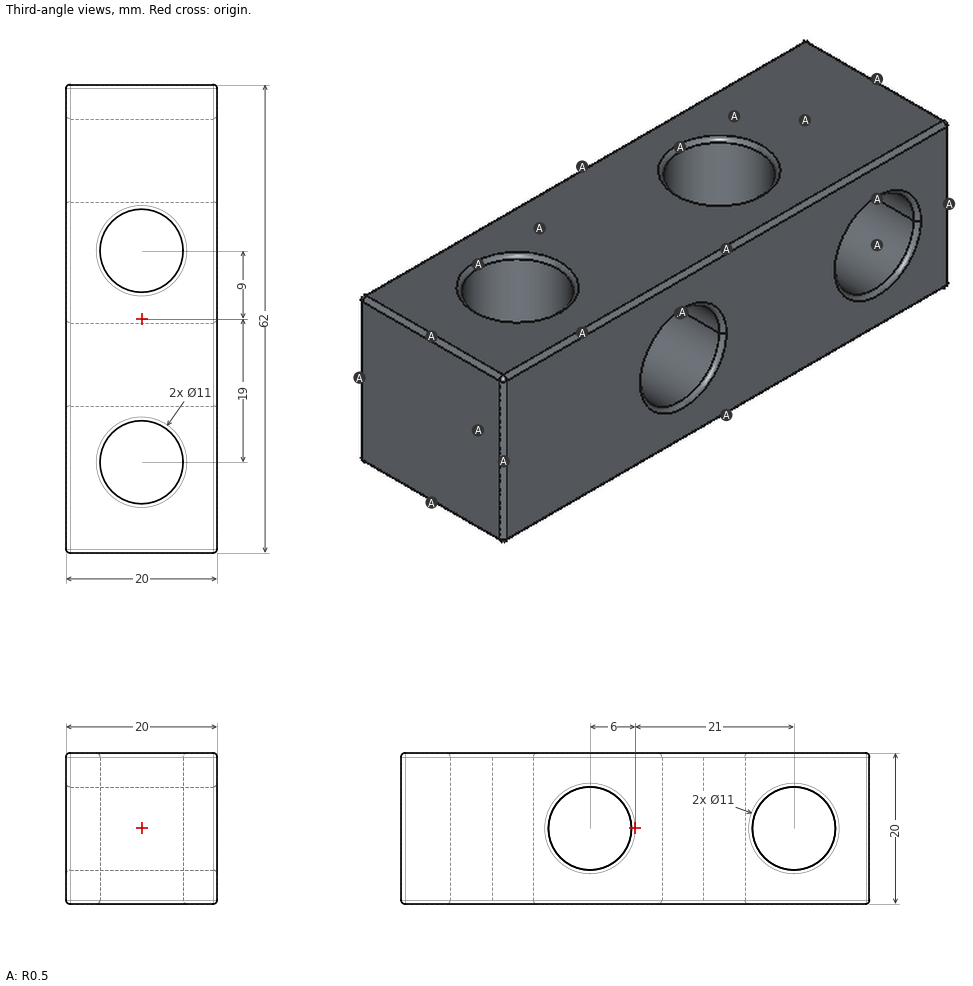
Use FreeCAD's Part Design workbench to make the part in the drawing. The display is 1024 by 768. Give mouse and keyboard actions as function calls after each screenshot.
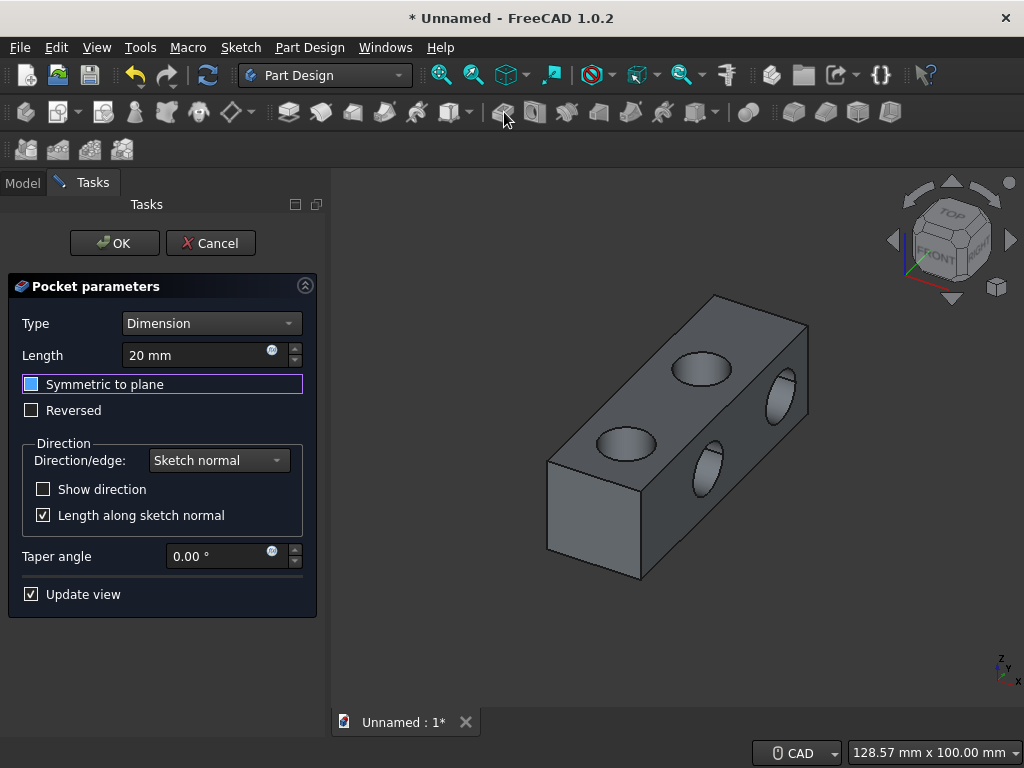
click(115, 243)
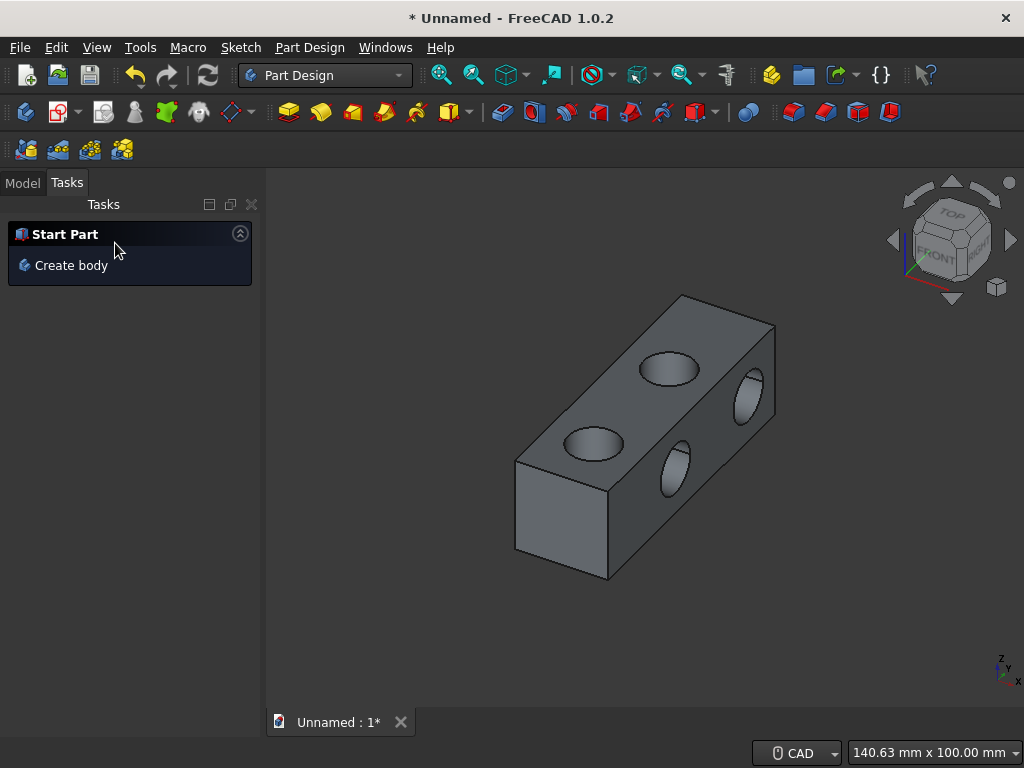
click(716, 416)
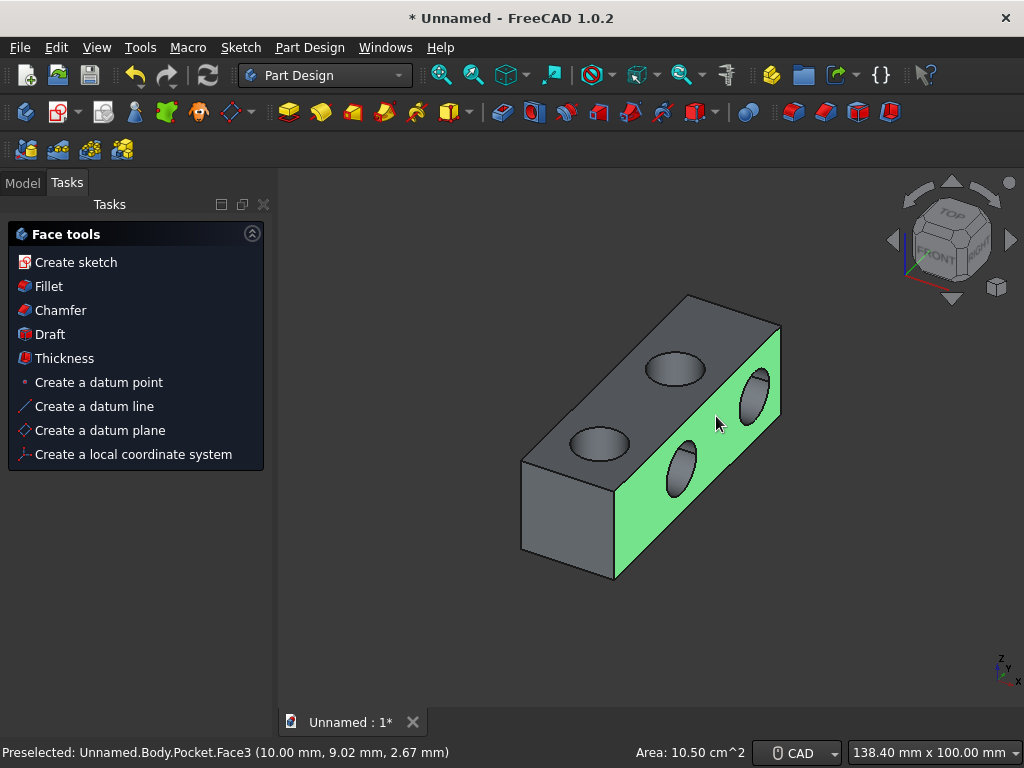
click(640, 420, ctrl)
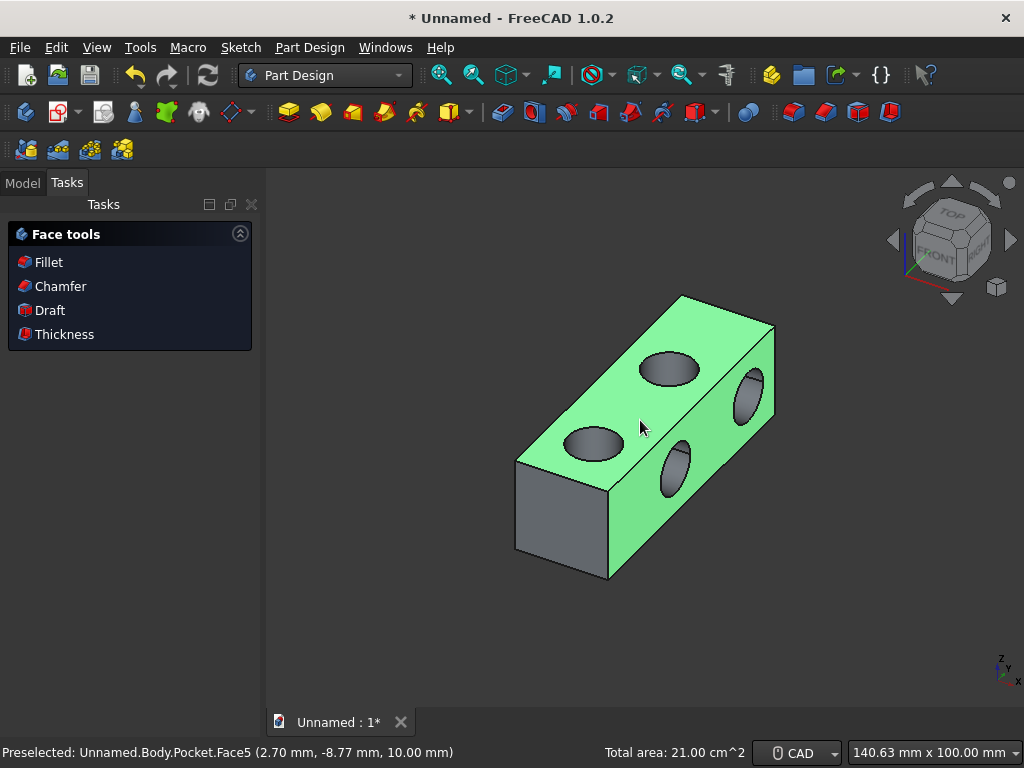
key(0)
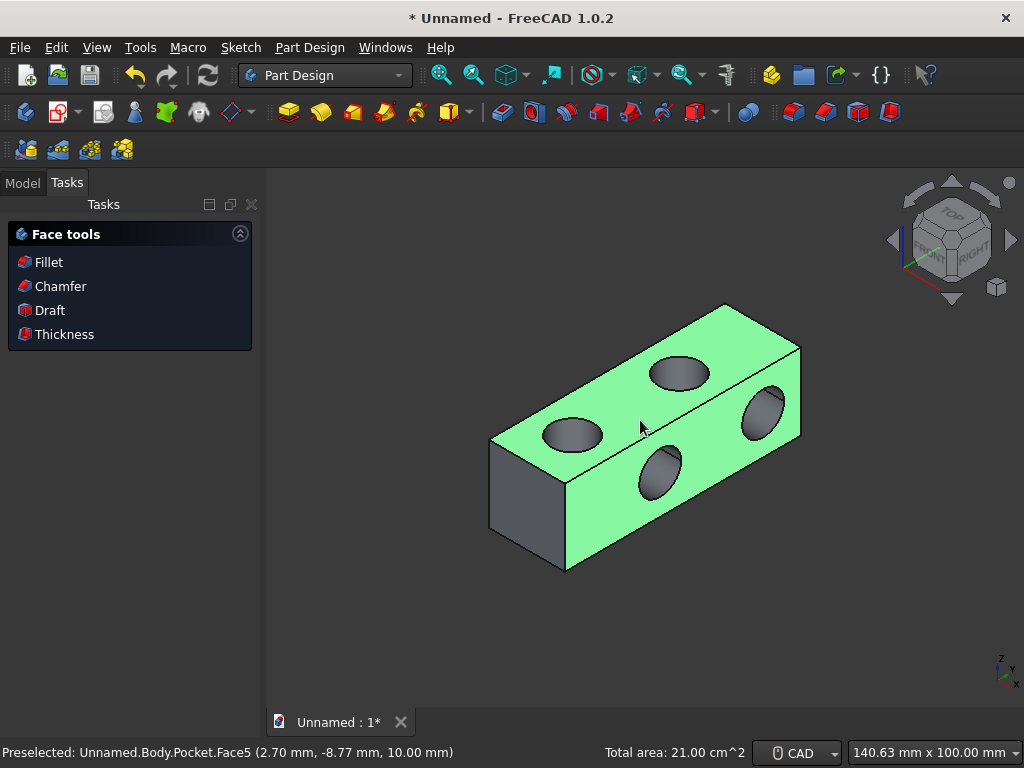
key(2)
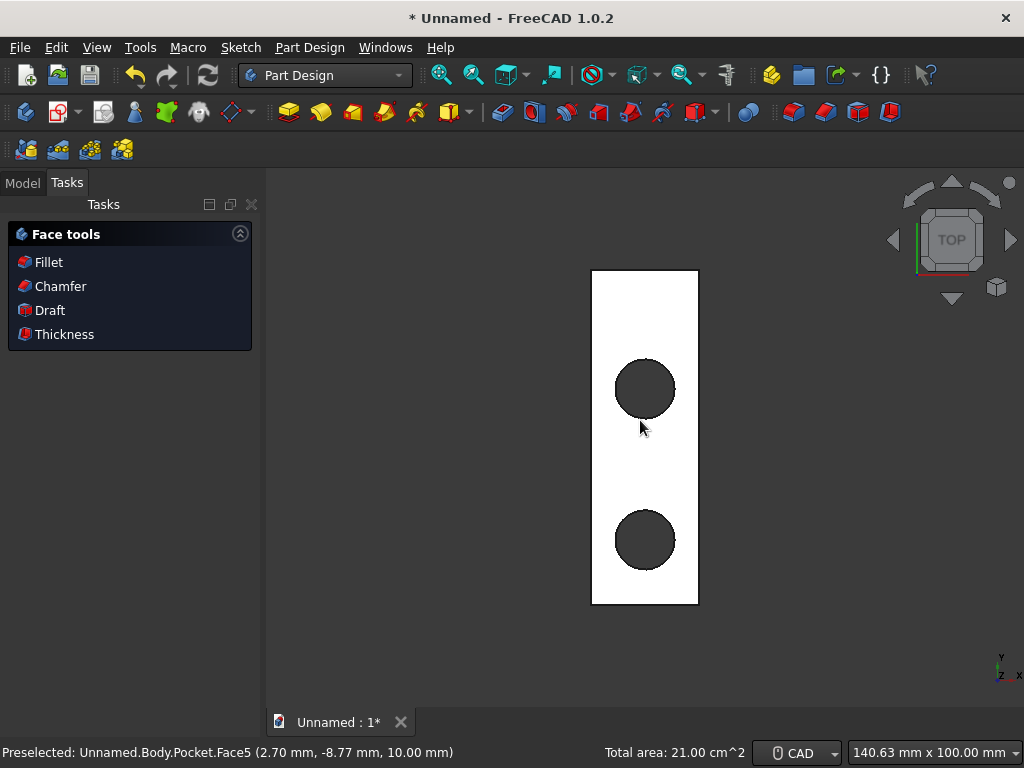
key(1)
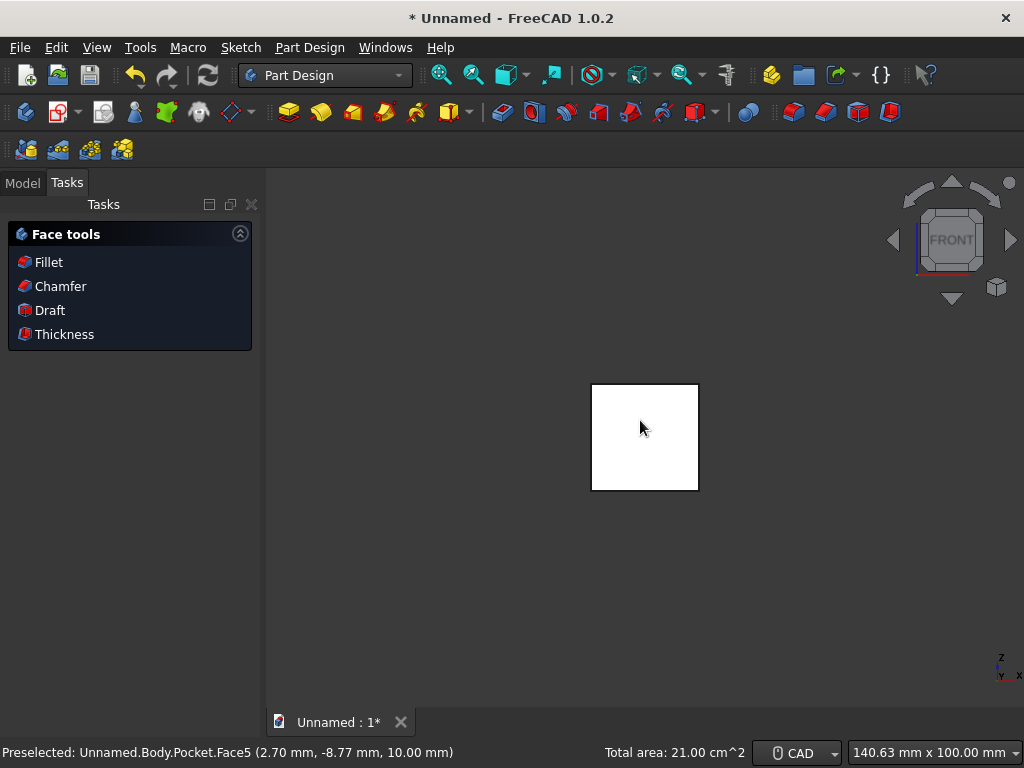
key(v)
key(f)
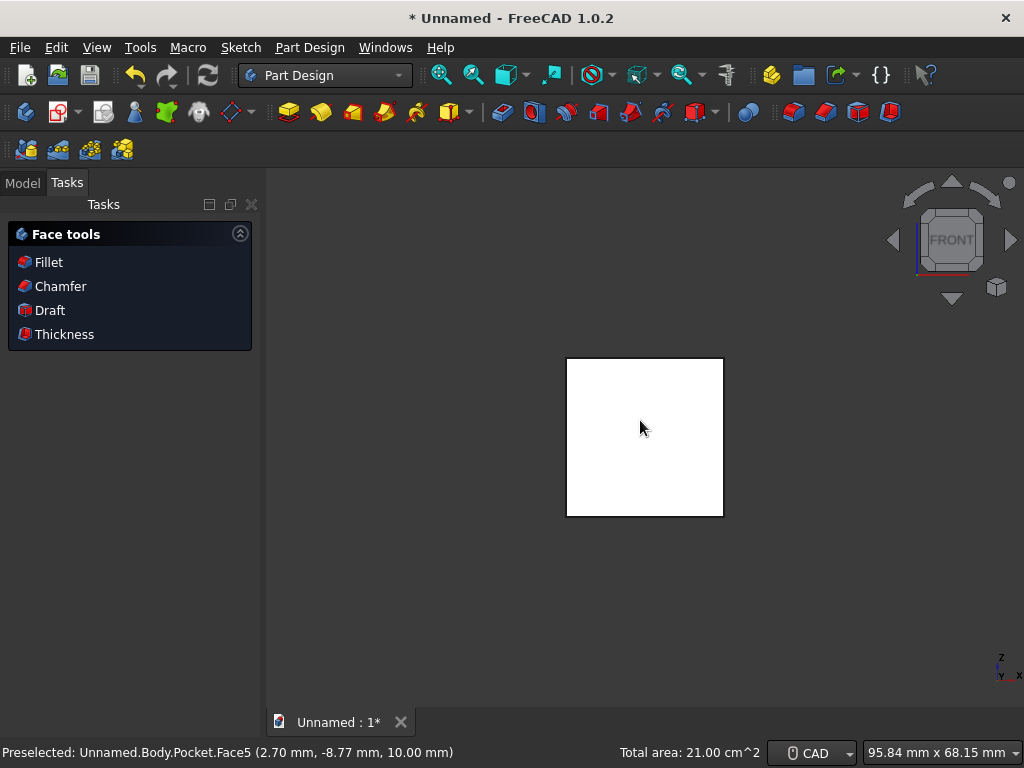
key(3)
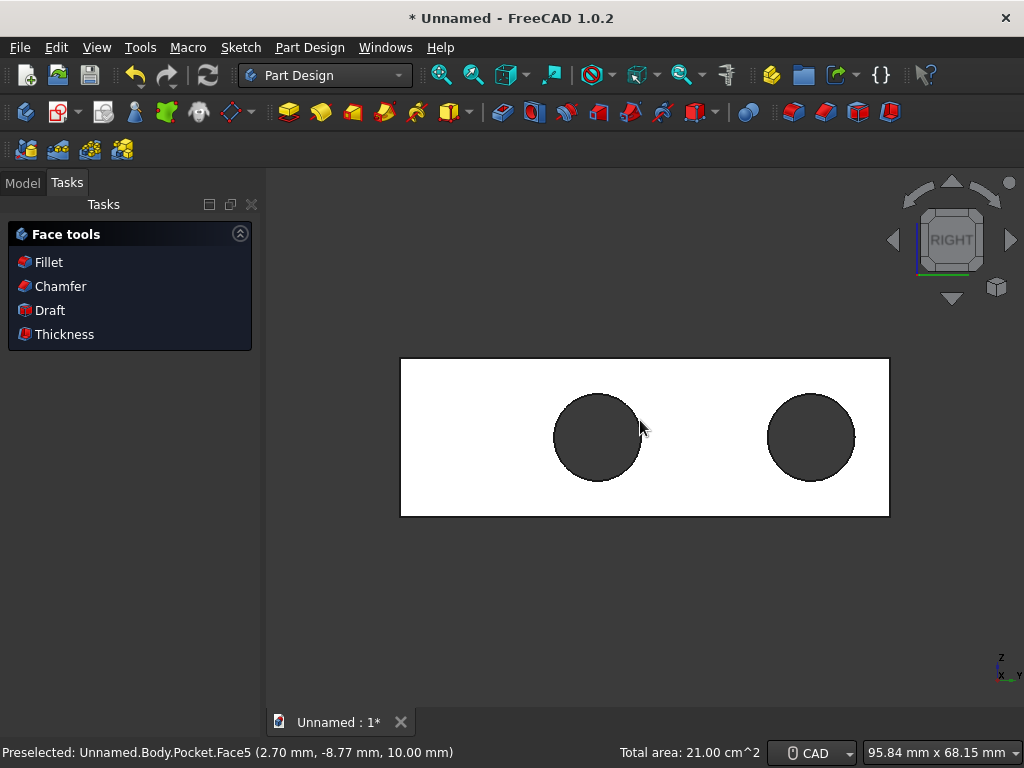
key(5)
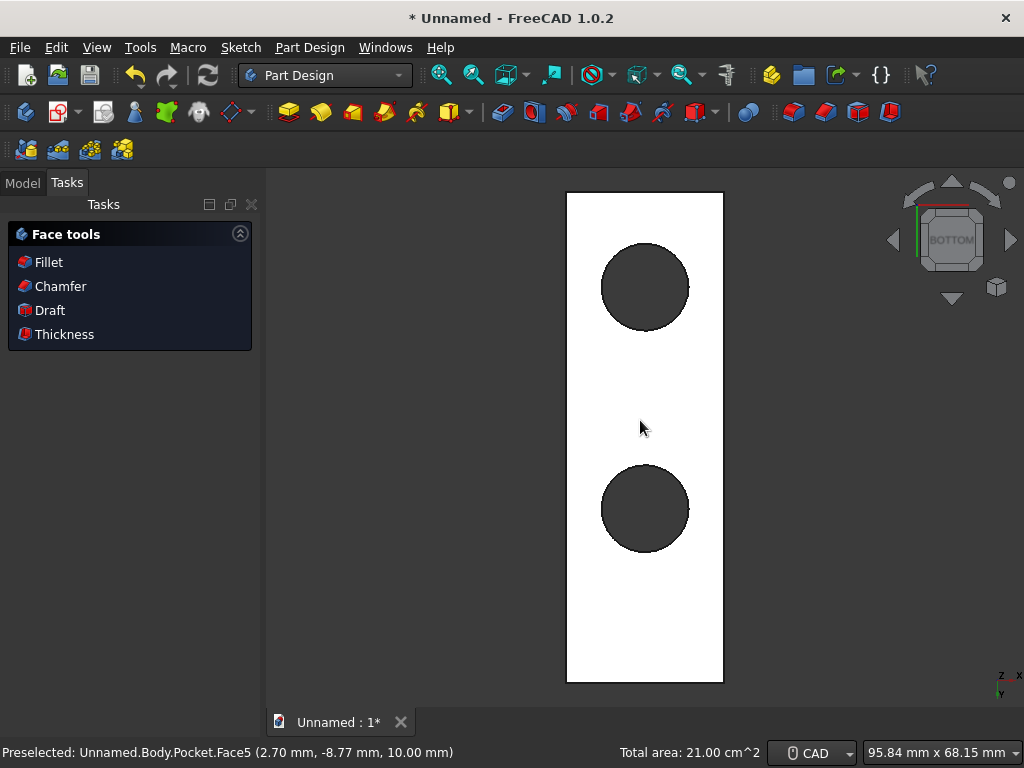
click(668, 366, ctrl)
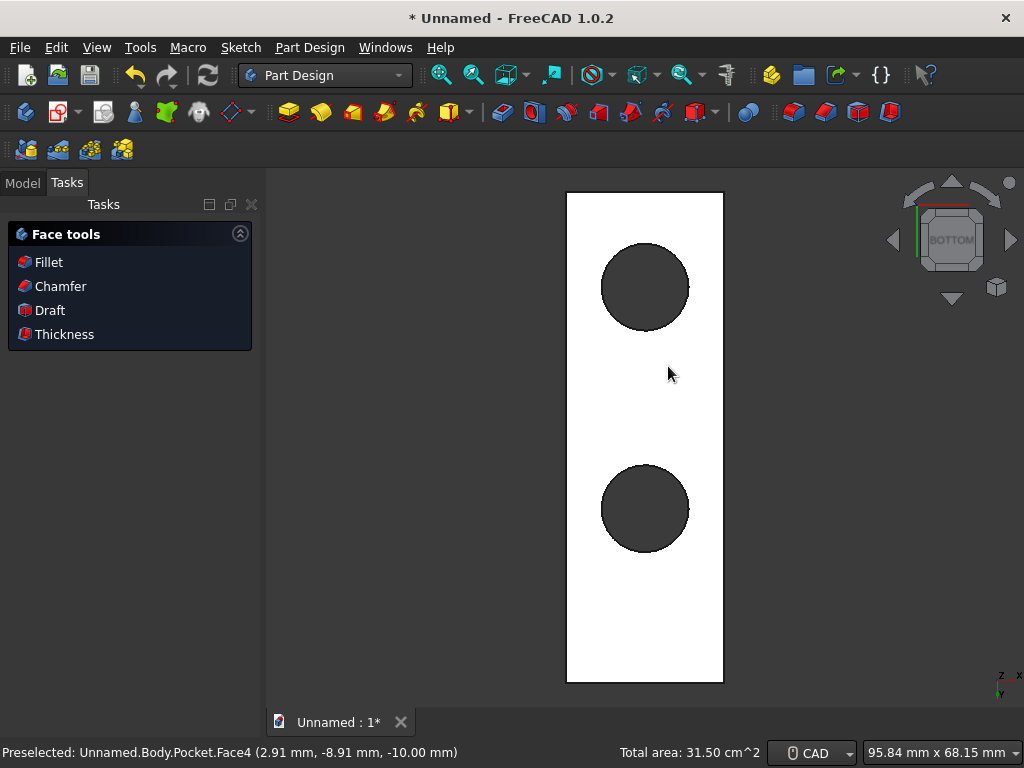
key(4)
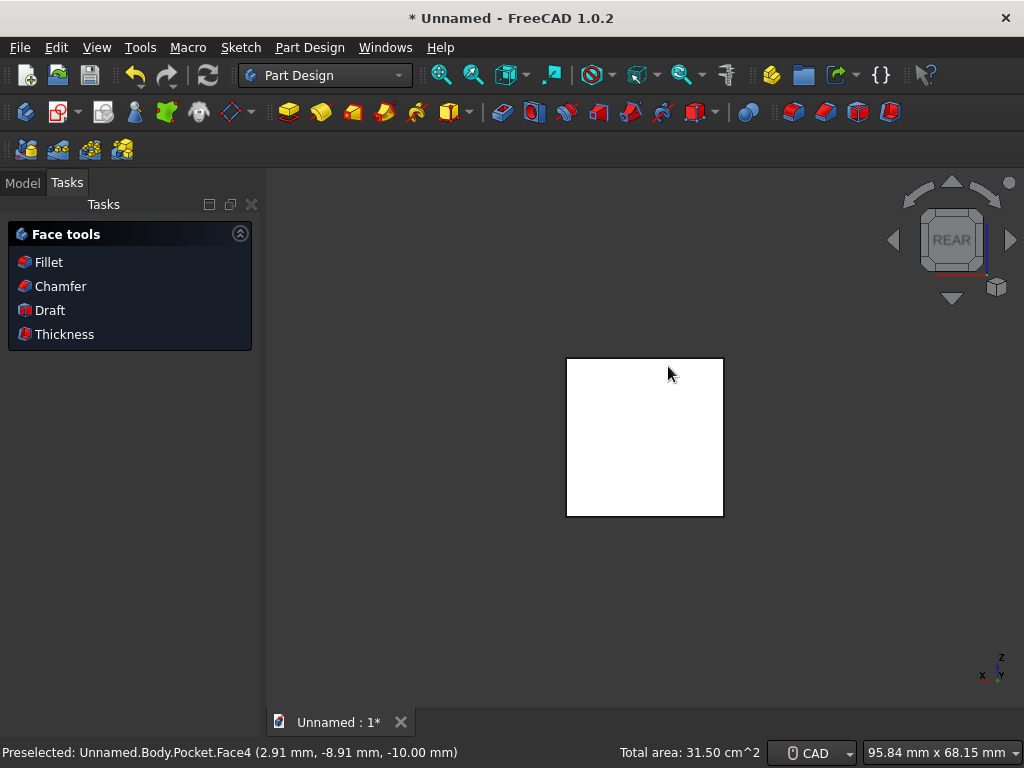
click(442, 76)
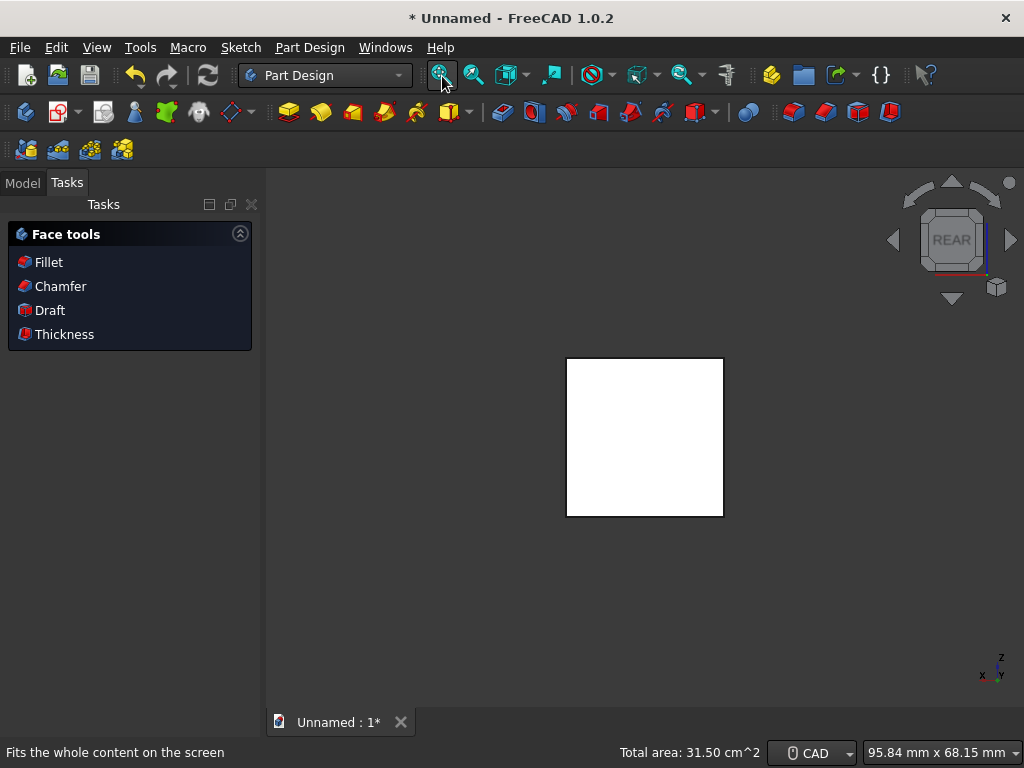
key(6)